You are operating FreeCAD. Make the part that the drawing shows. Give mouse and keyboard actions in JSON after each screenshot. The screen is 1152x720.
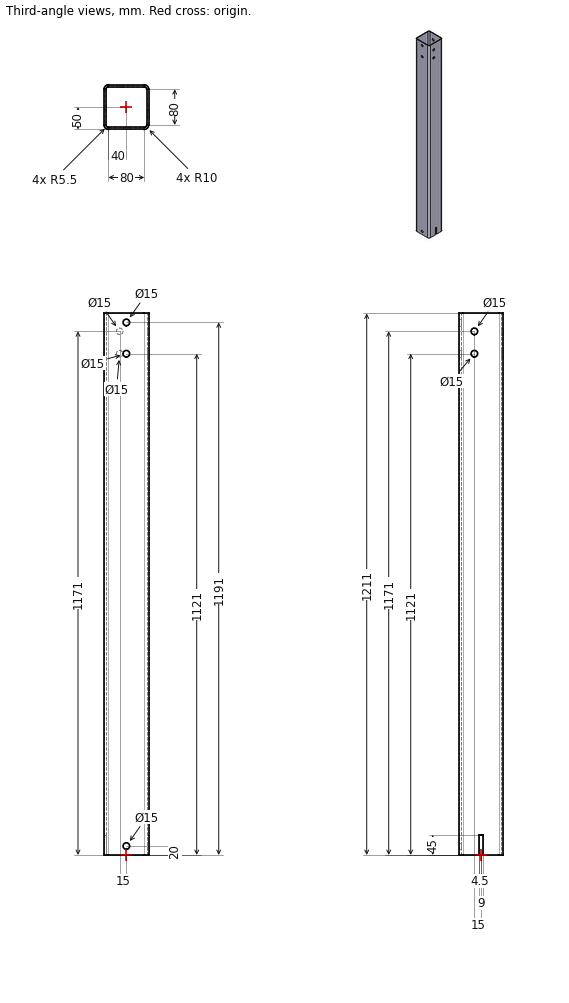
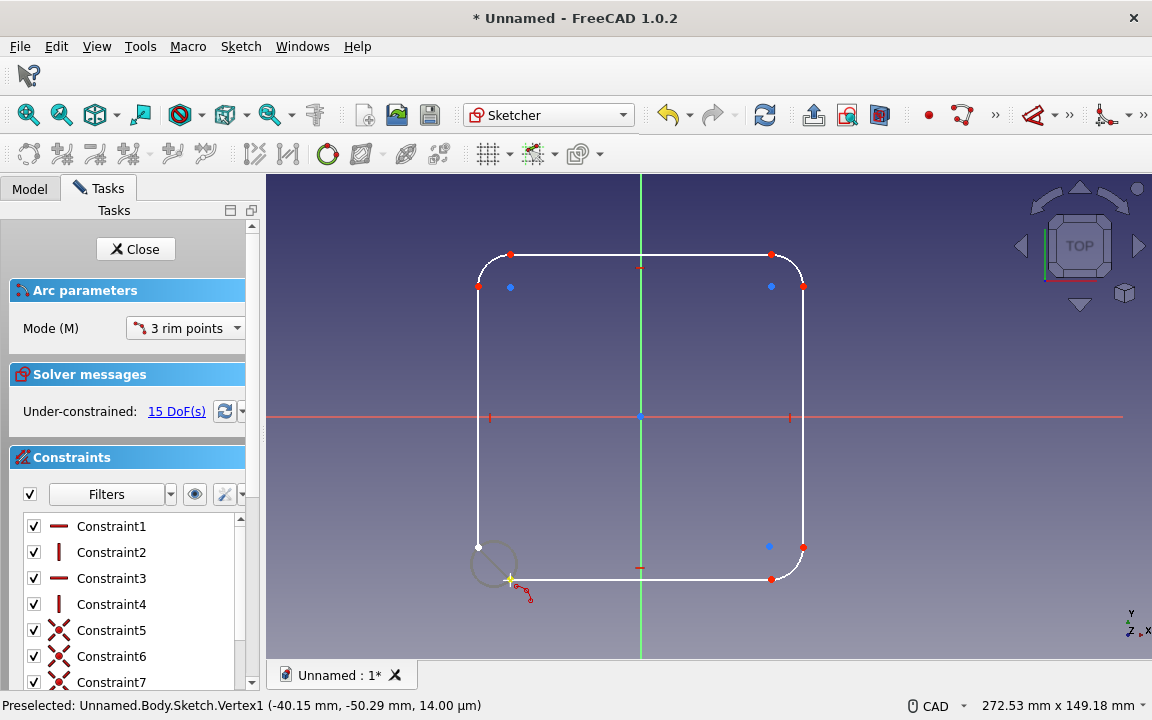
{"action": "scroll", "coordinate": [487, 570], "scroll_direction": "up", "scroll_amount": 3}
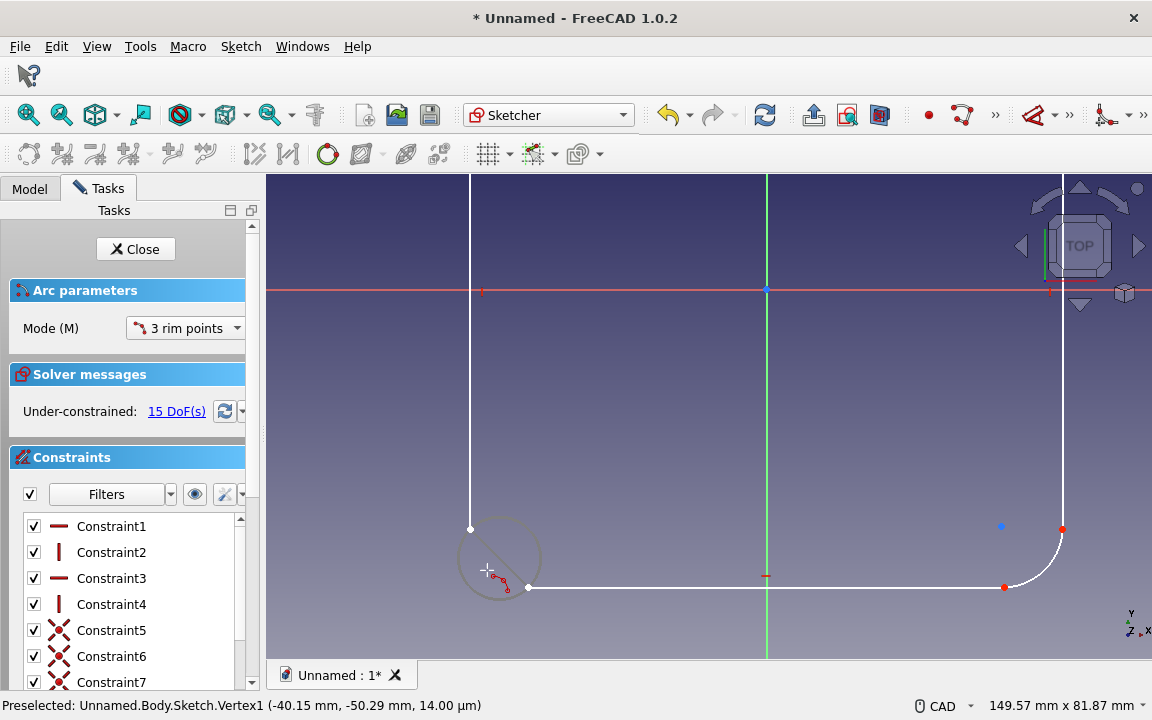
{"action": "left_click", "coordinate": [488, 568]}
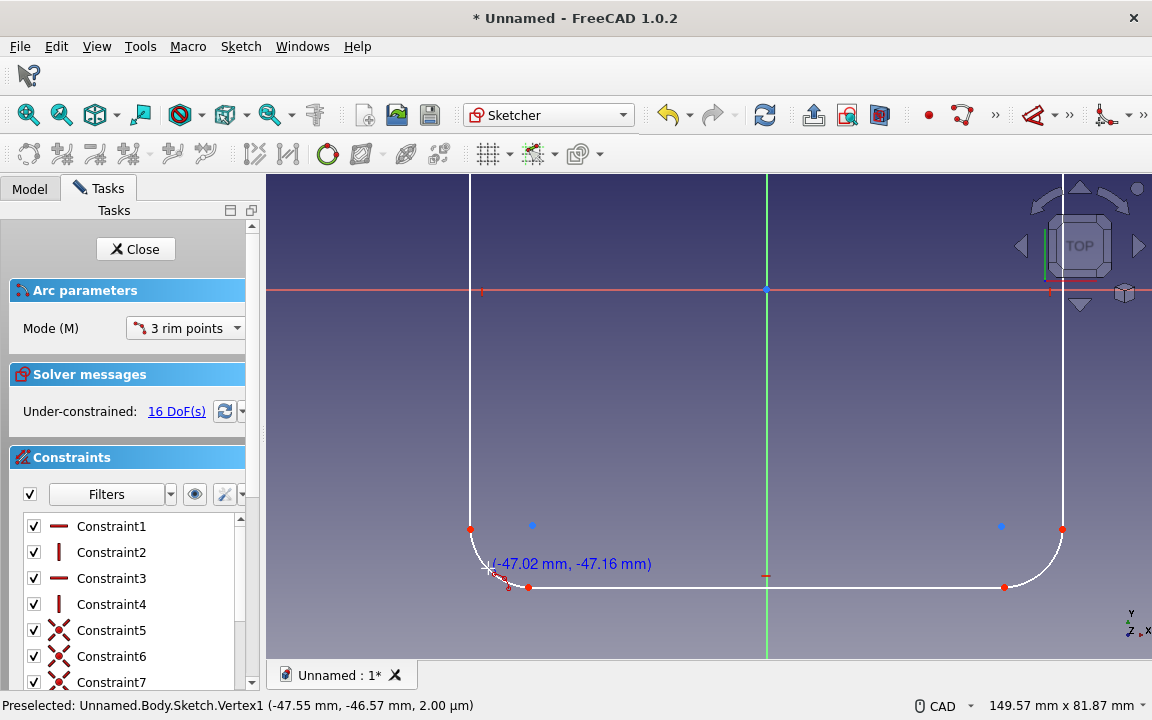
{"action": "key", "text": "g l"}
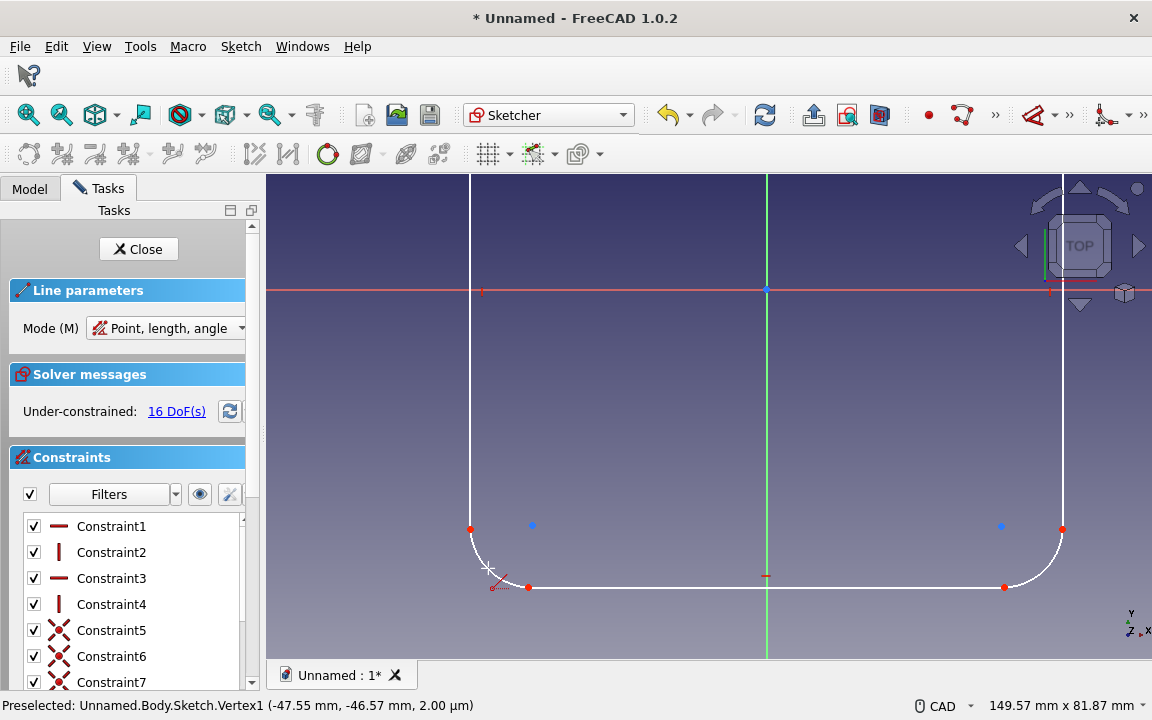
{"action": "scroll", "coordinate": [487, 571], "scroll_direction": "down", "scroll_amount": 3}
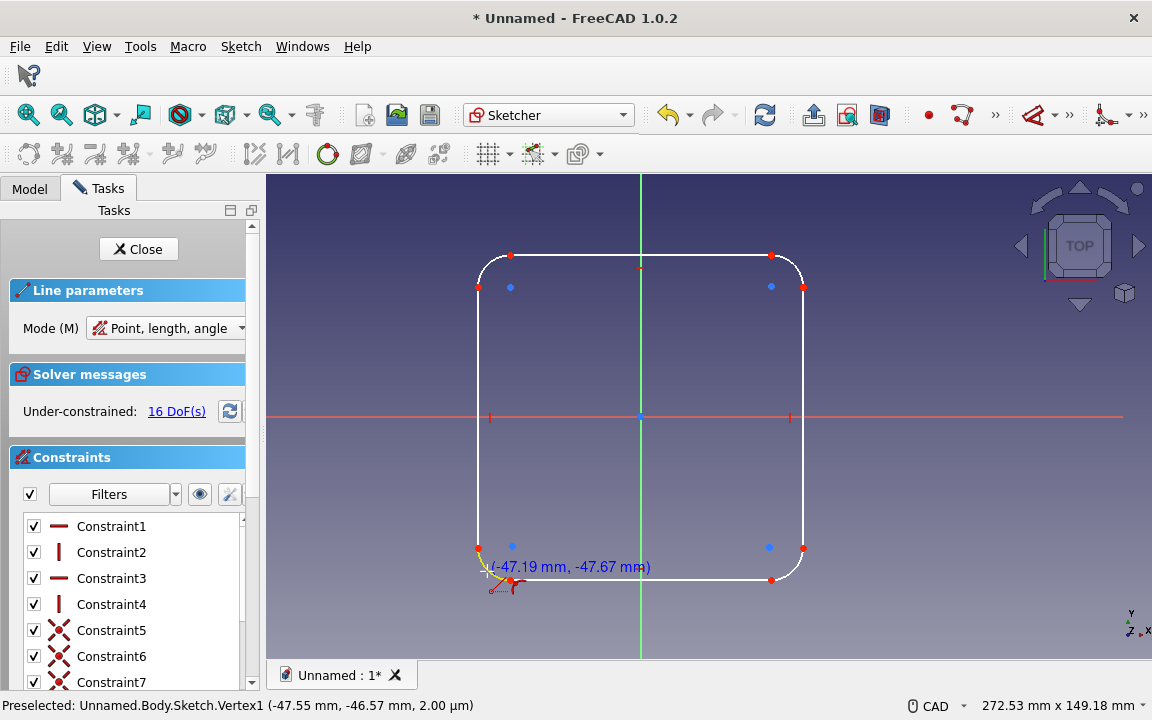
{"action": "left_click", "coordinate": [771, 565]}
{"action": "left_click", "coordinate": [510, 565]}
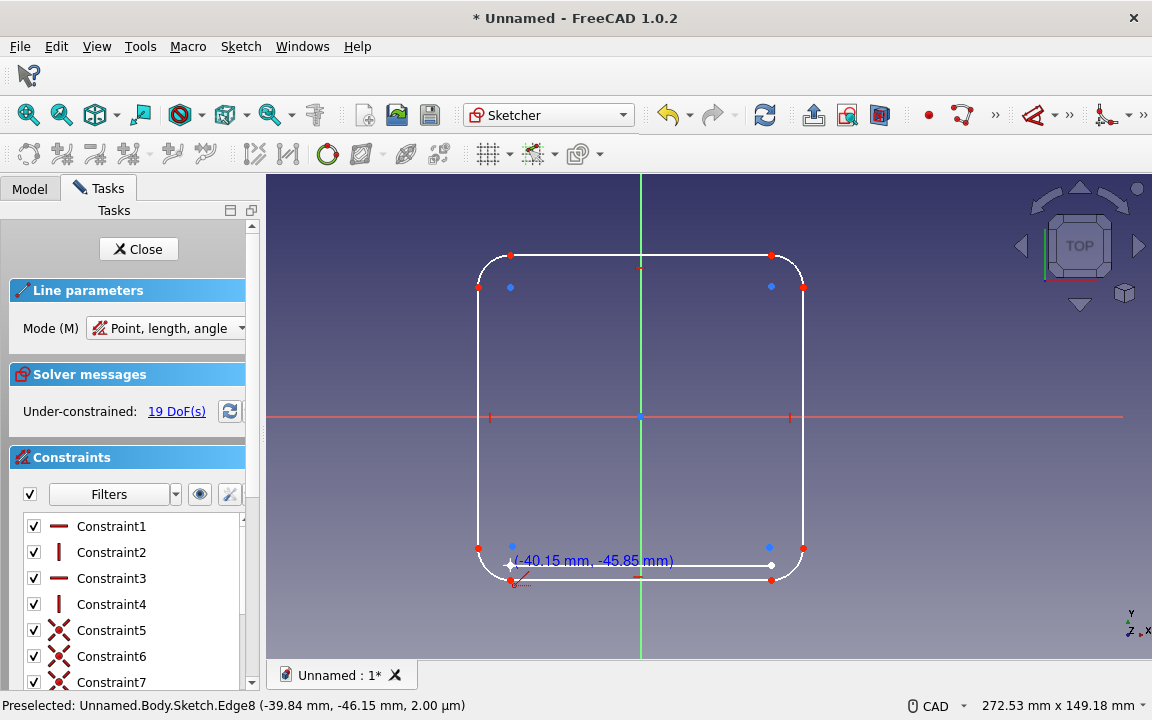
{"action": "left_click", "coordinate": [493, 547]}
{"action": "left_click", "coordinate": [493, 287]}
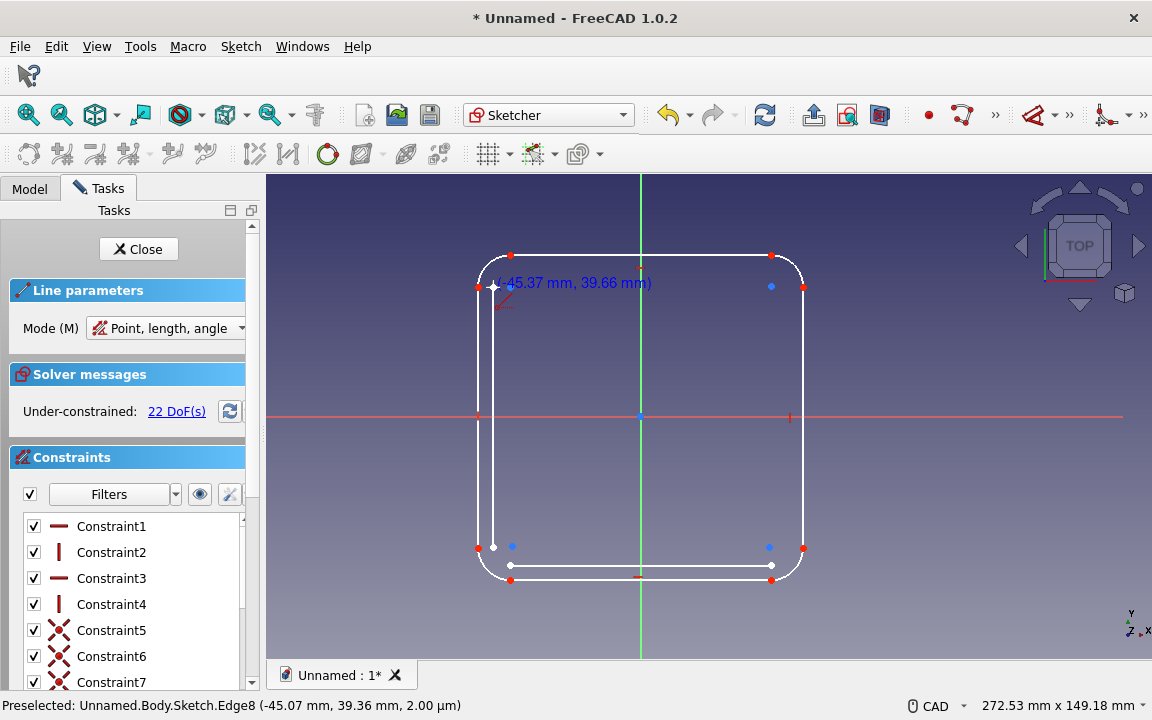
{"action": "left_click", "coordinate": [510, 269]}
{"action": "left_click", "coordinate": [771, 269]}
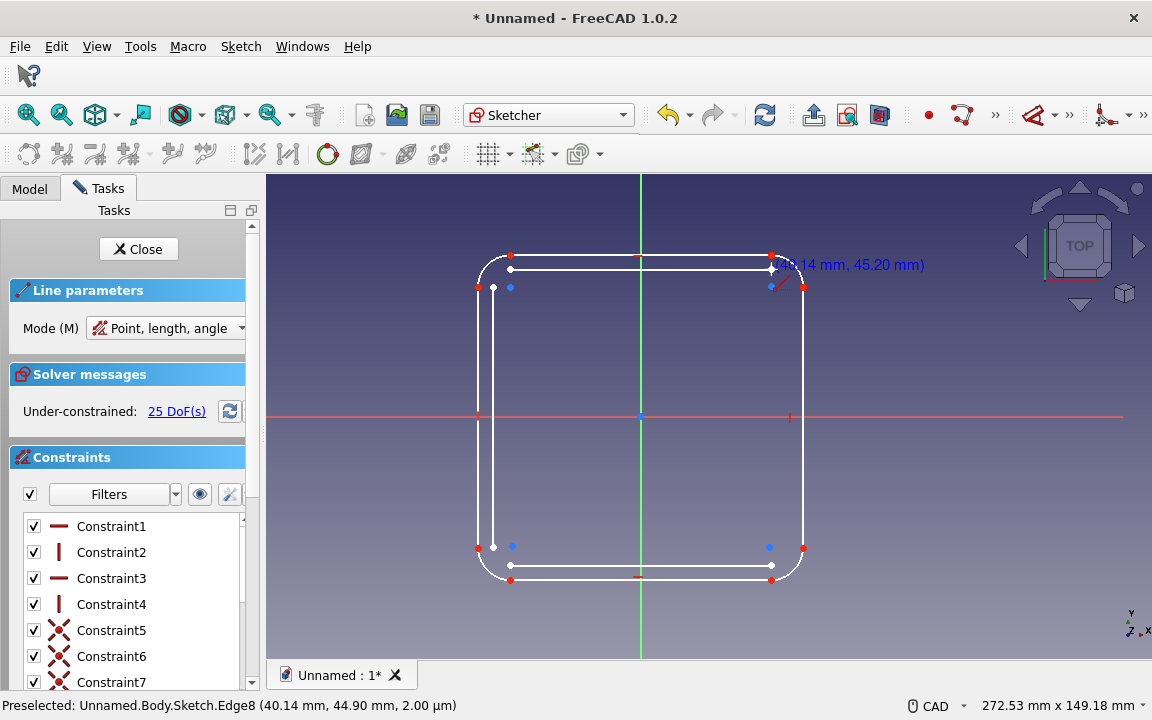
{"action": "left_click", "coordinate": [788, 287]}
{"action": "left_click", "coordinate": [788, 547]}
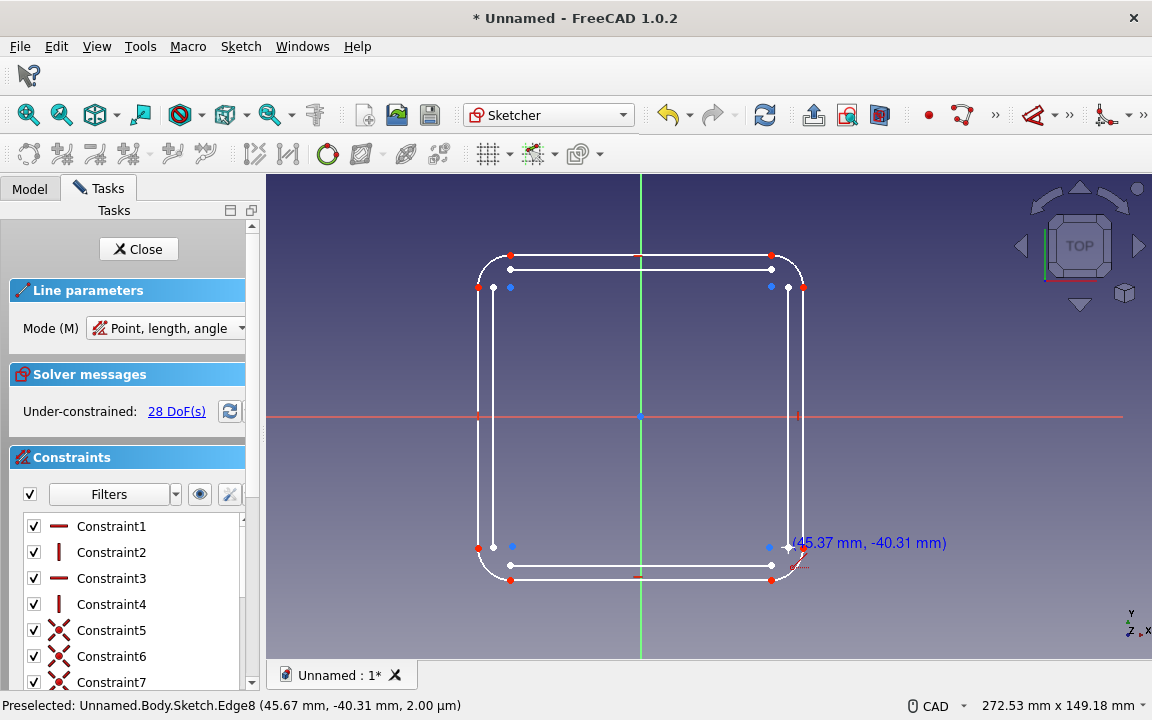
{"action": "key", "text": "g 3 a"}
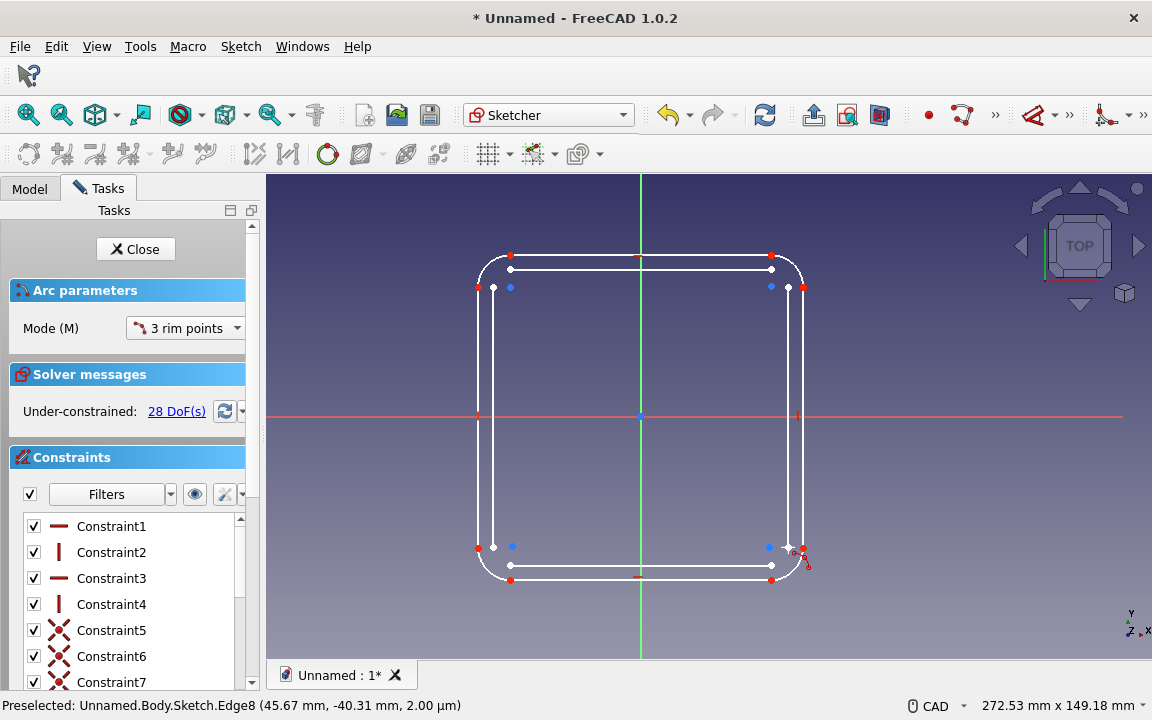
{"action": "left_click", "coordinate": [510, 566]}
{"action": "left_click", "coordinate": [493, 548]}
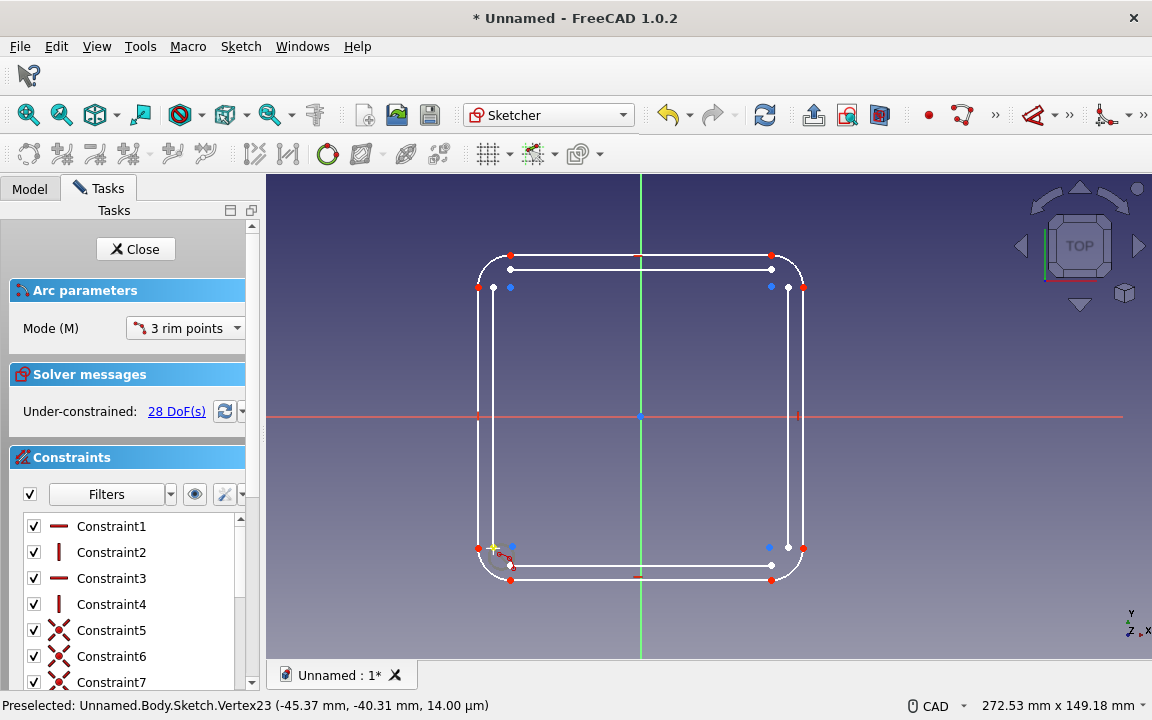
{"action": "scroll", "coordinate": [498, 560], "scroll_direction": "up", "scroll_amount": 6}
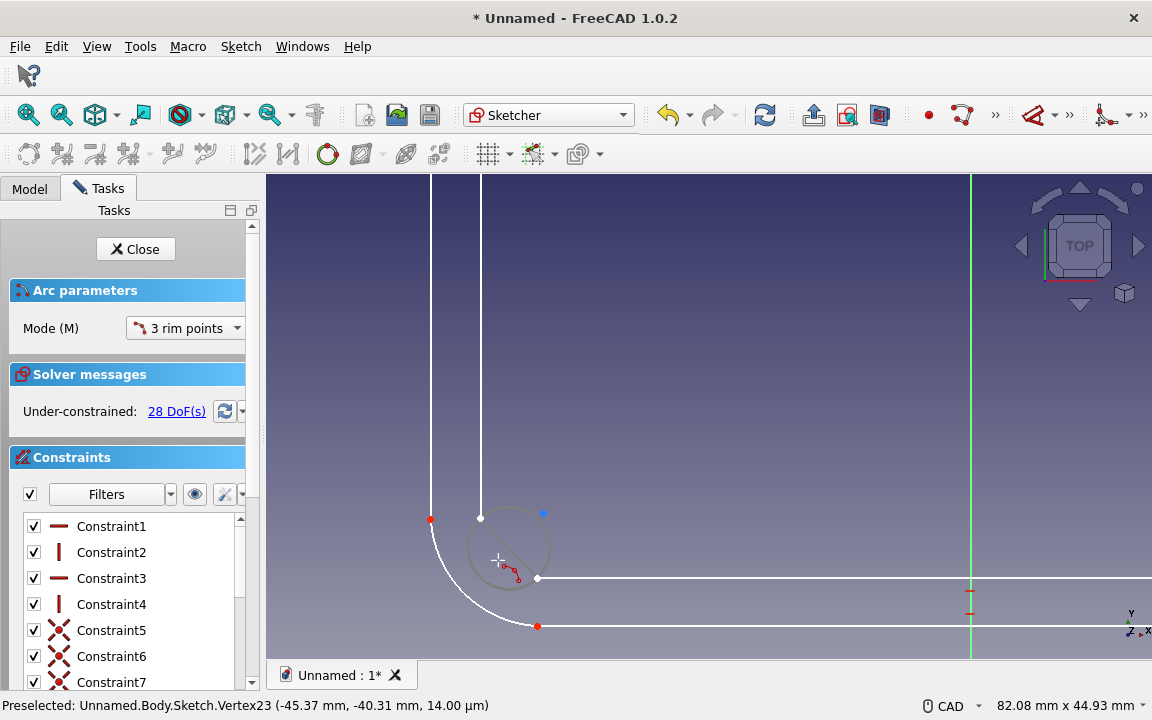
{"action": "left_click", "coordinate": [497, 557]}